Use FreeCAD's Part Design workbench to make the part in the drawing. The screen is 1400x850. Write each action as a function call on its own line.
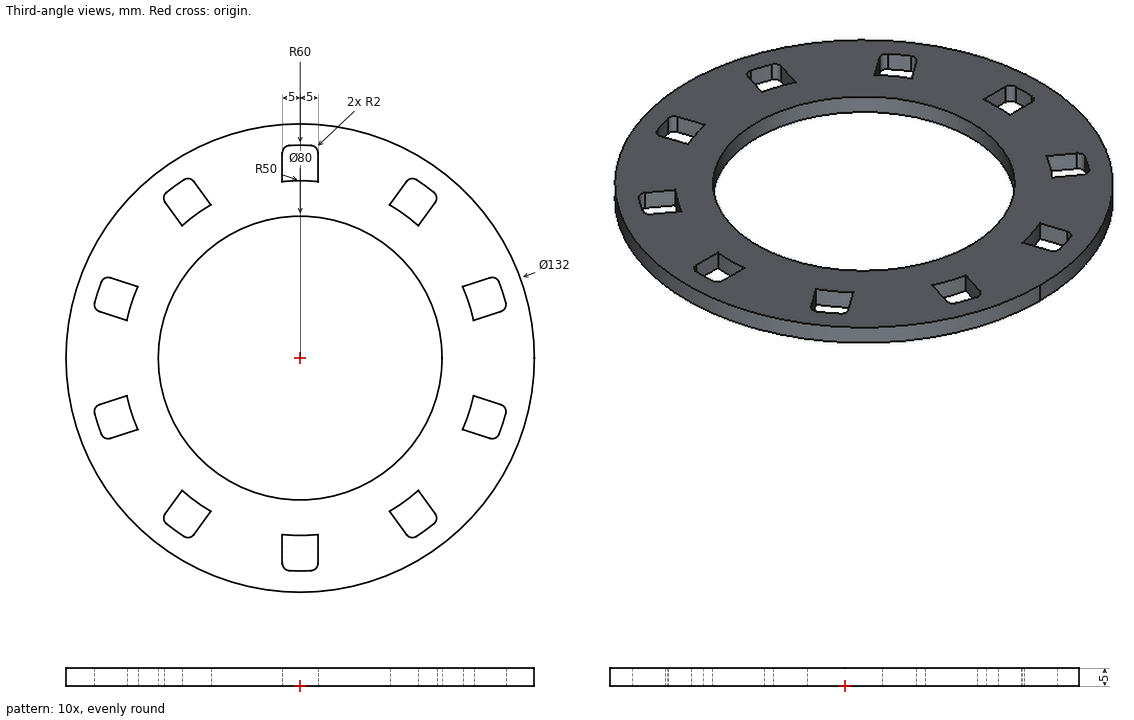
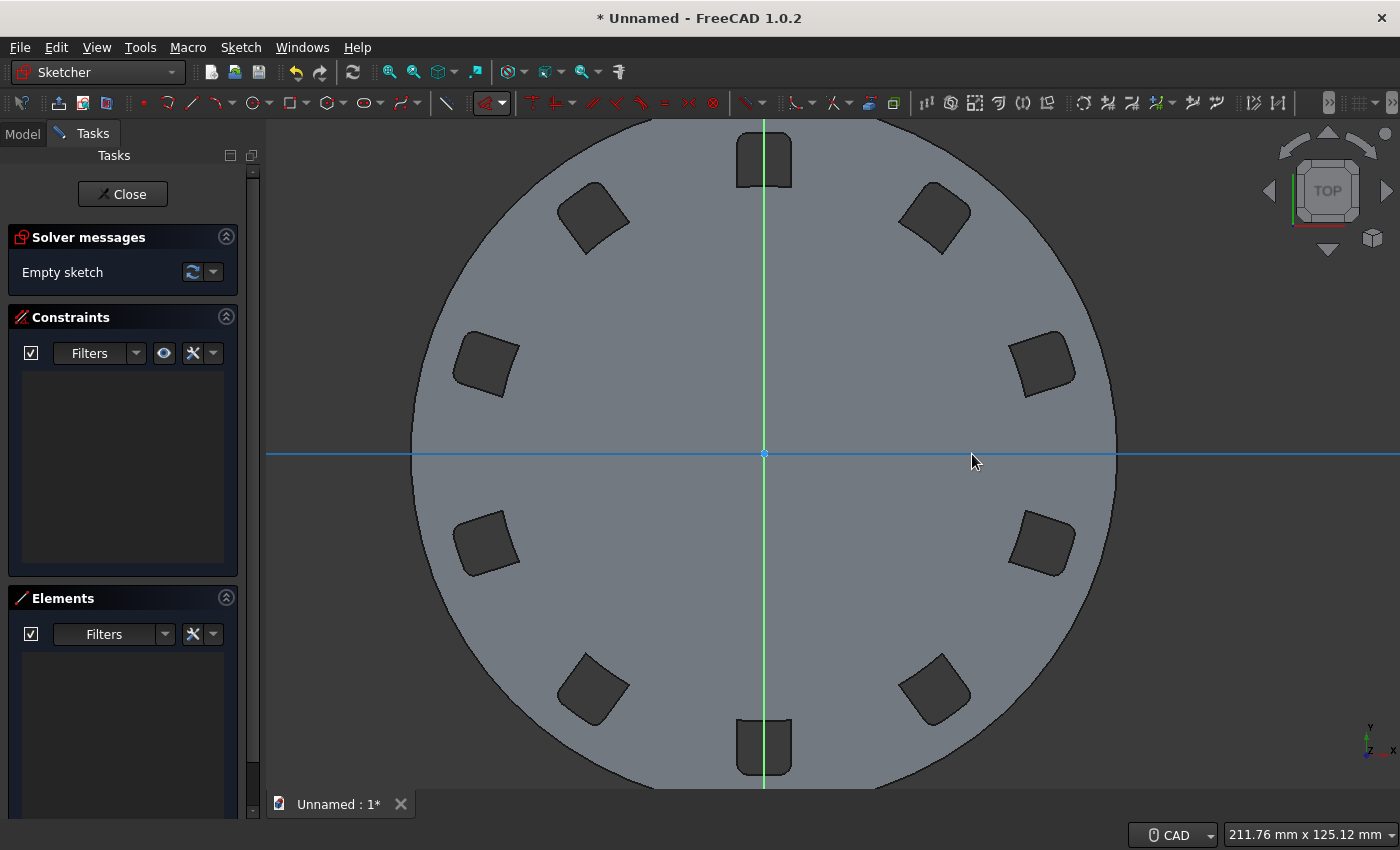
key(g)
key(c)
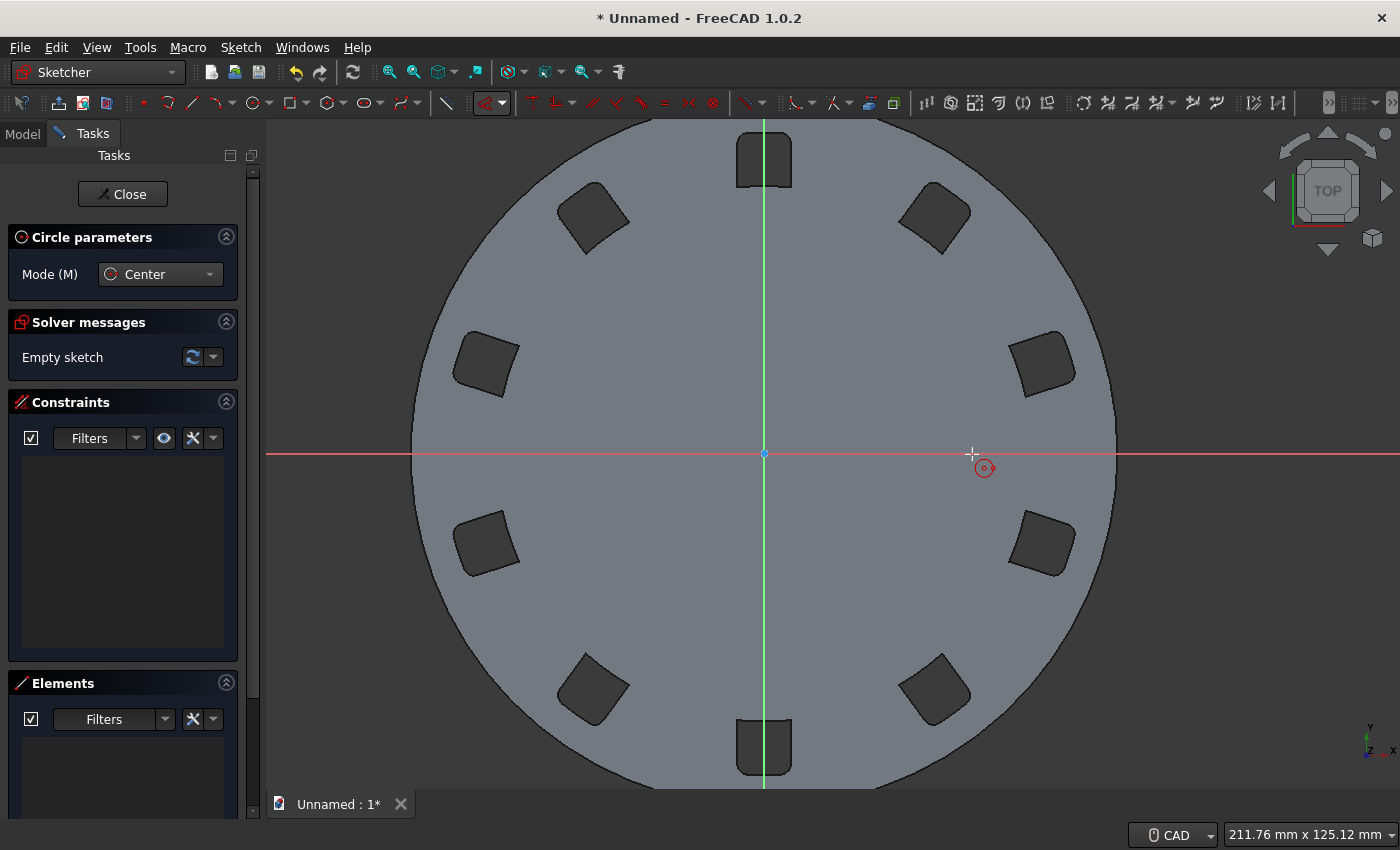
click(764, 454)
move(916, 302)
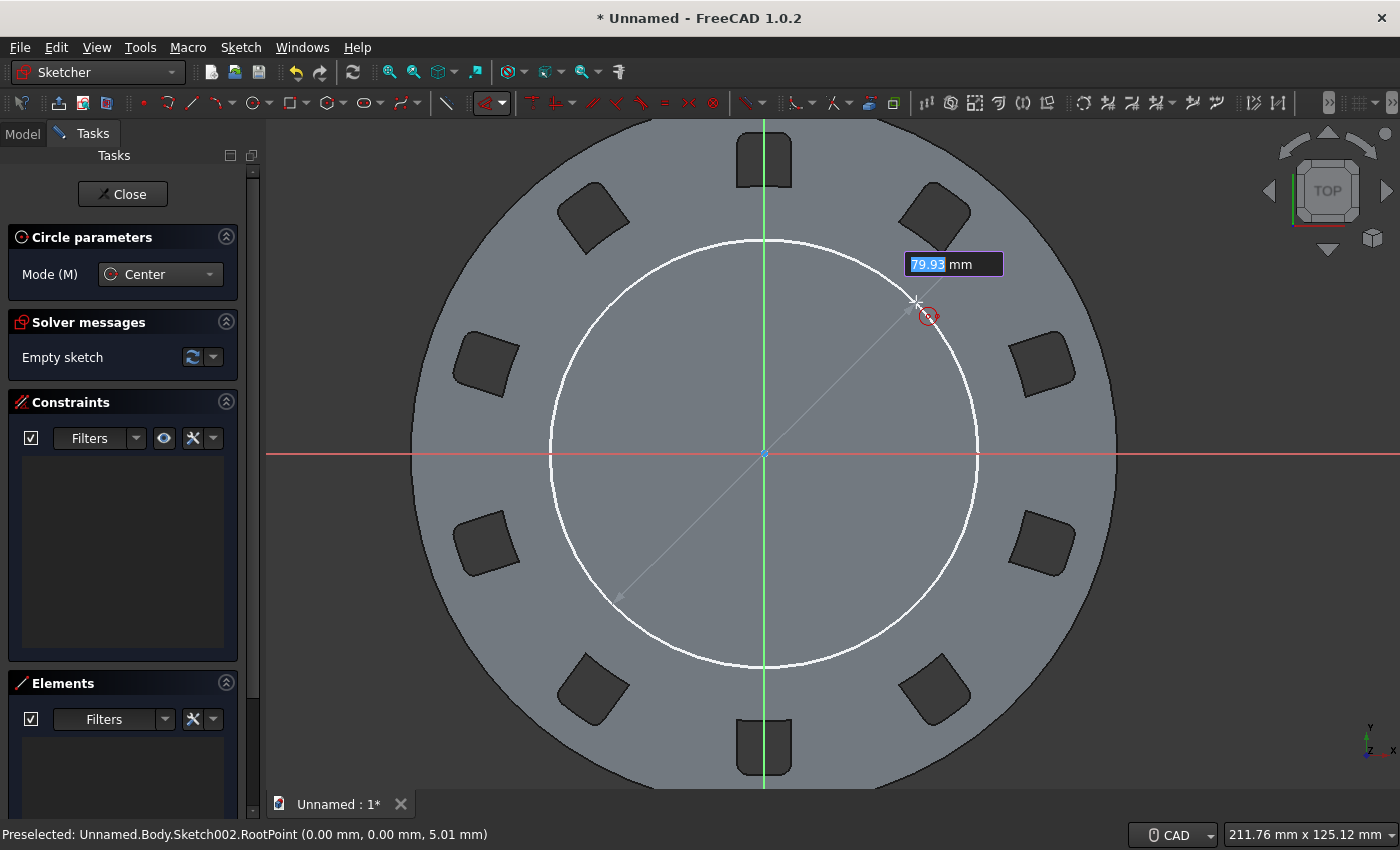
text(80)
key(Return)
key(Escape)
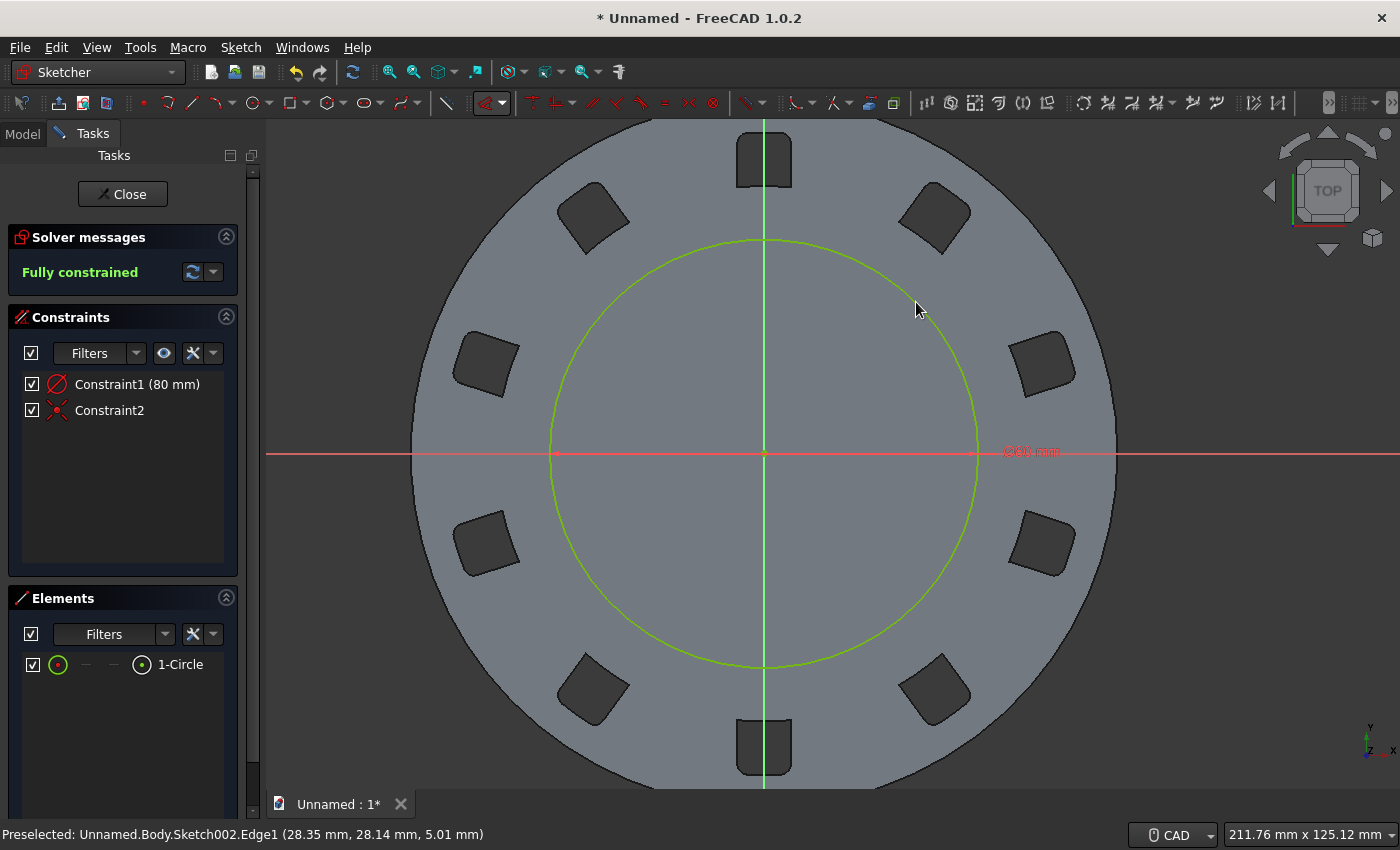
click(123, 194)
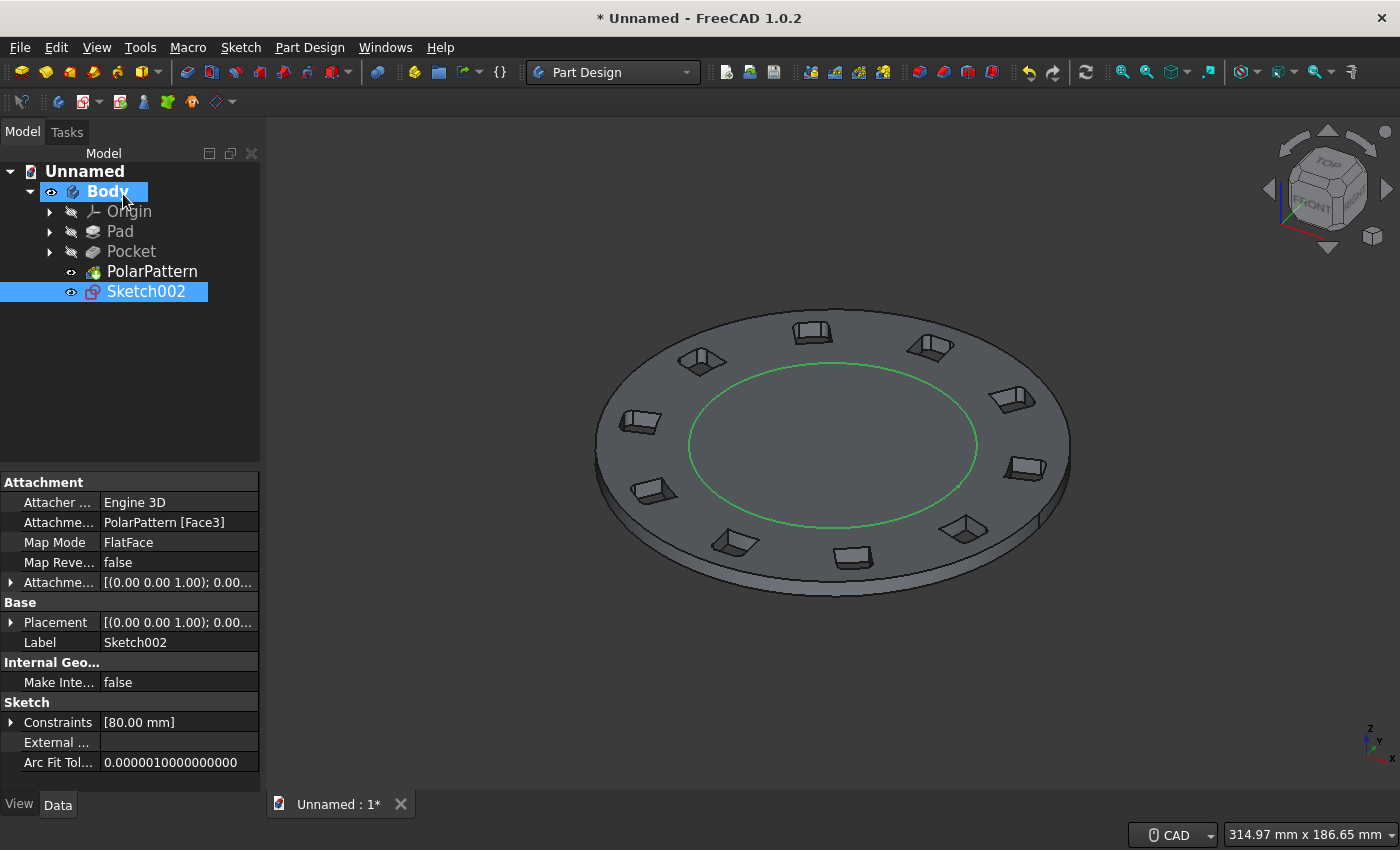
click(188, 72)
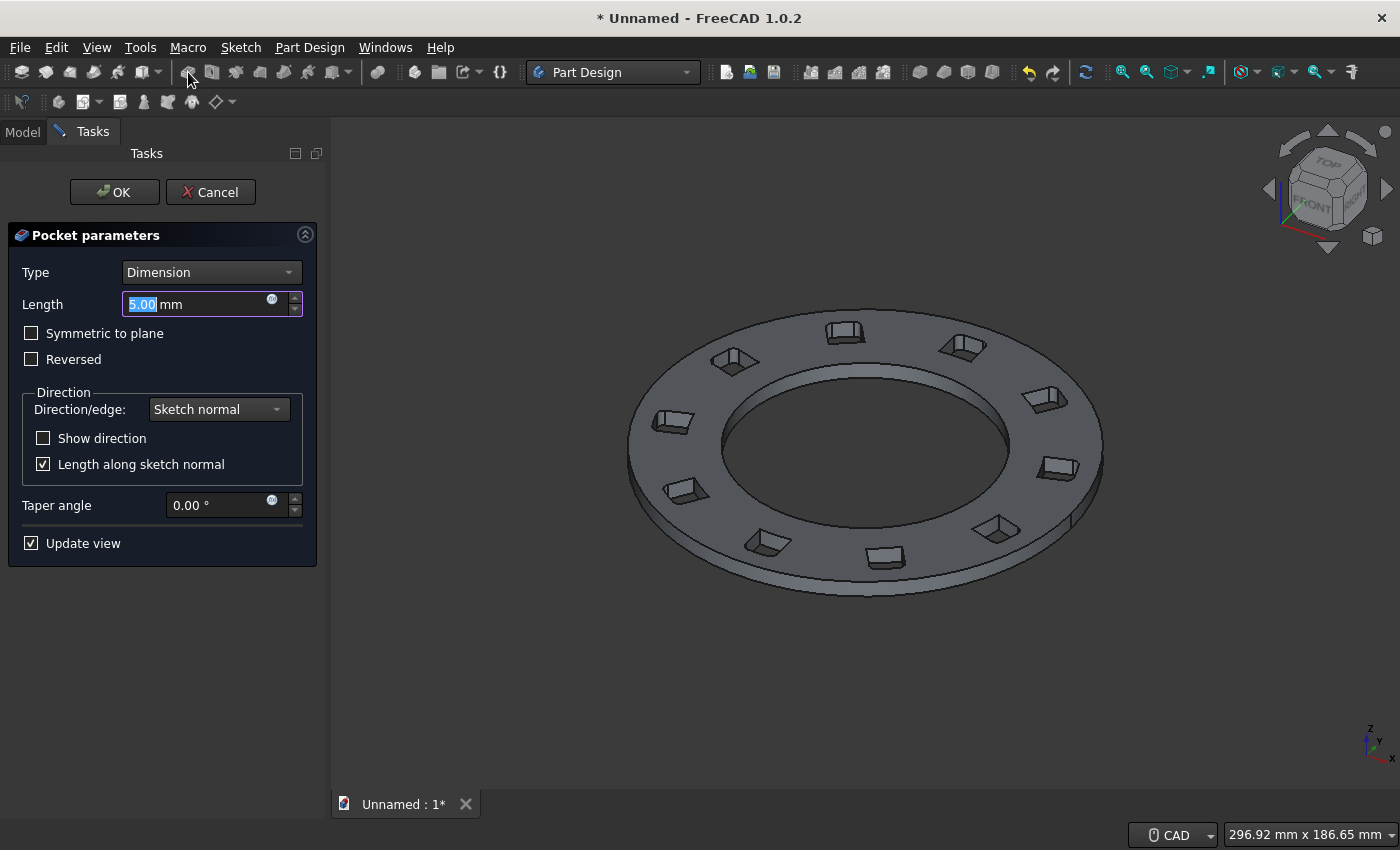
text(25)
key(Tab)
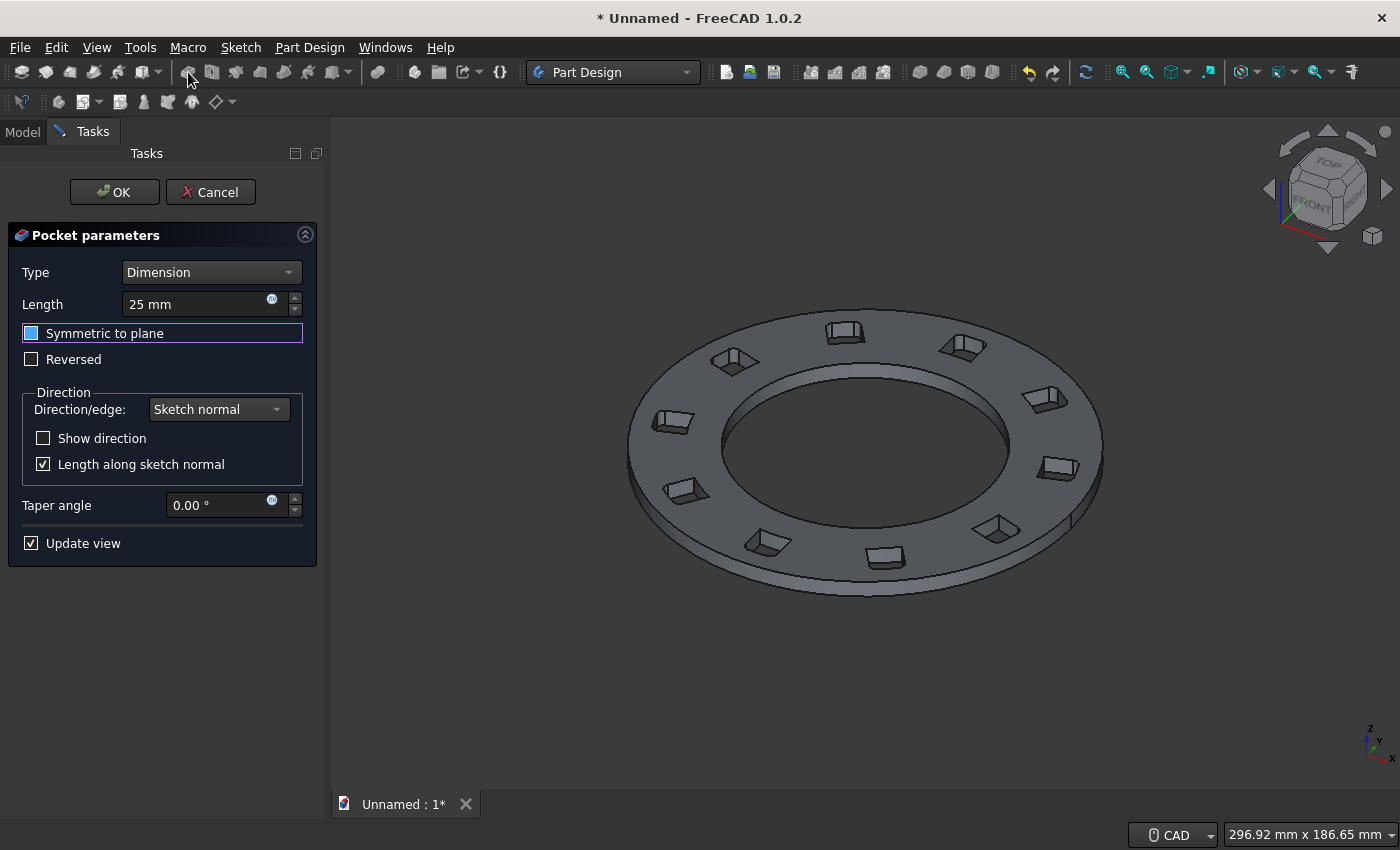
click(115, 192)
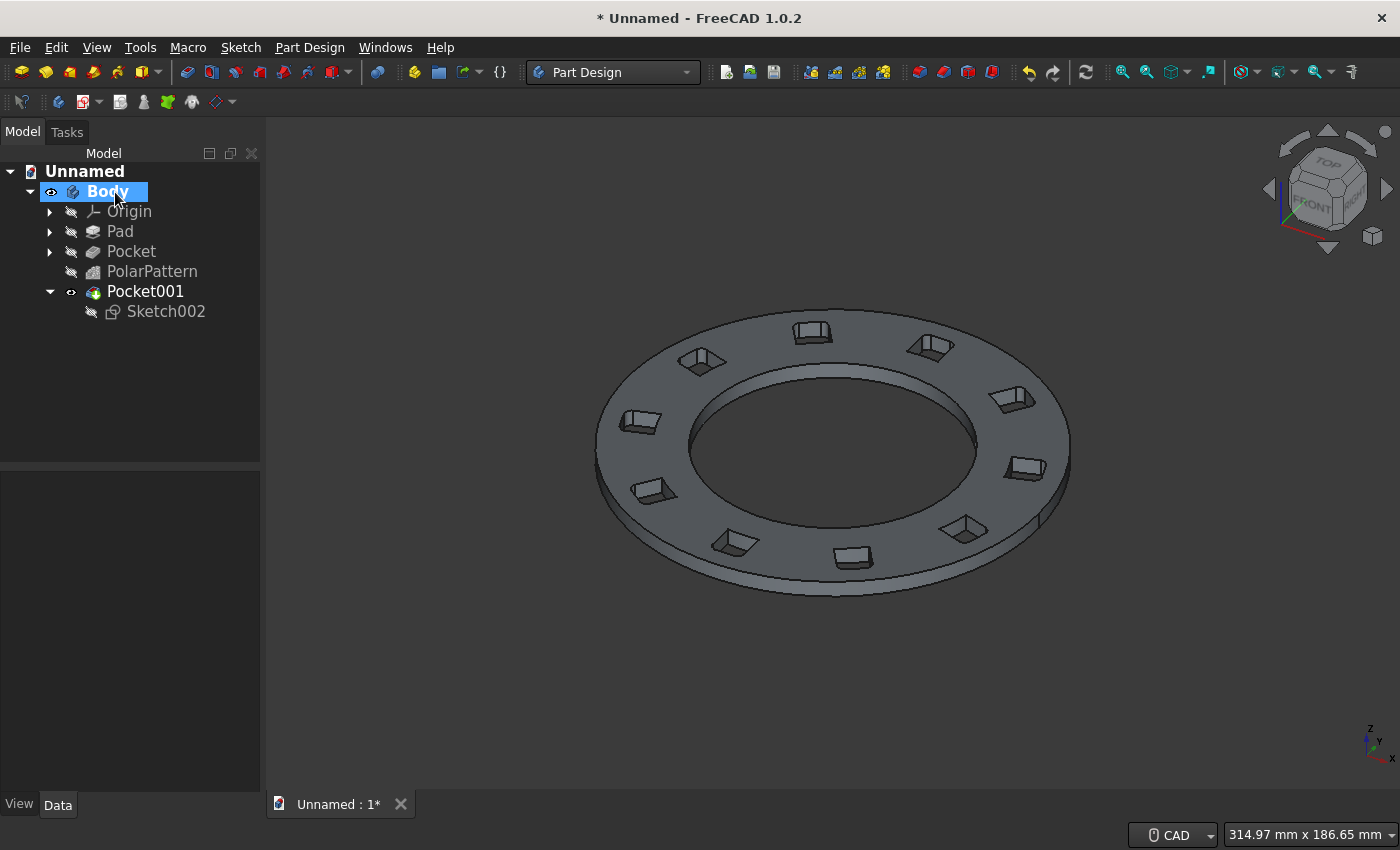
key(0)